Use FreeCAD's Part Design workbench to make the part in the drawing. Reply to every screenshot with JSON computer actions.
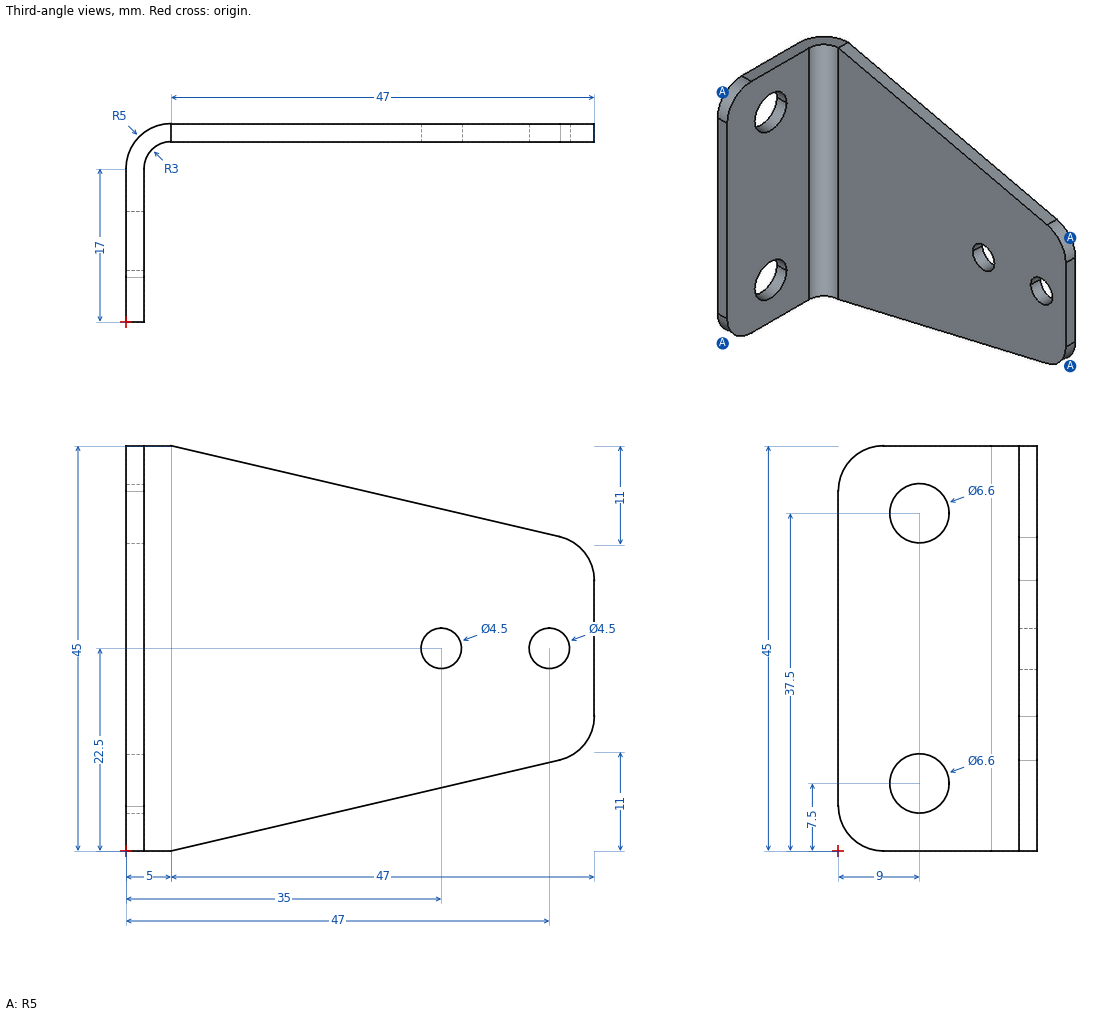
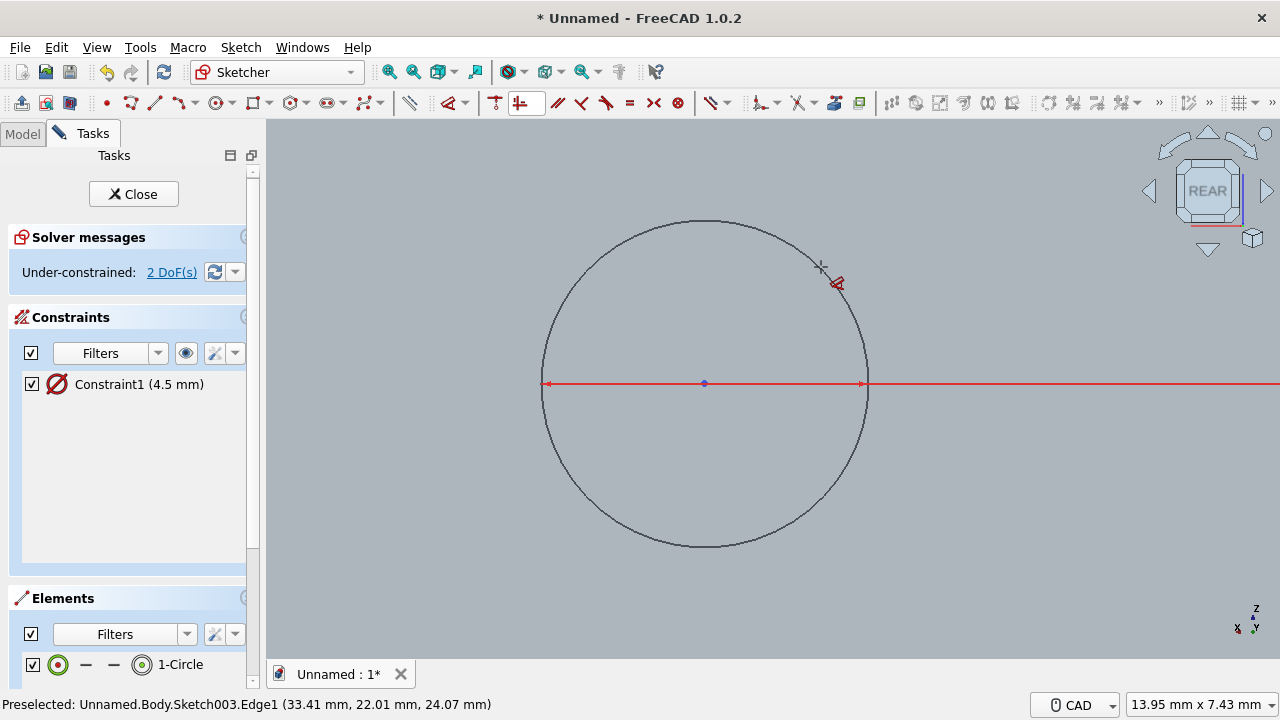
{"action": "left_click", "coordinate": [705, 384]}
{"action": "left_click", "coordinate": [910, 350]}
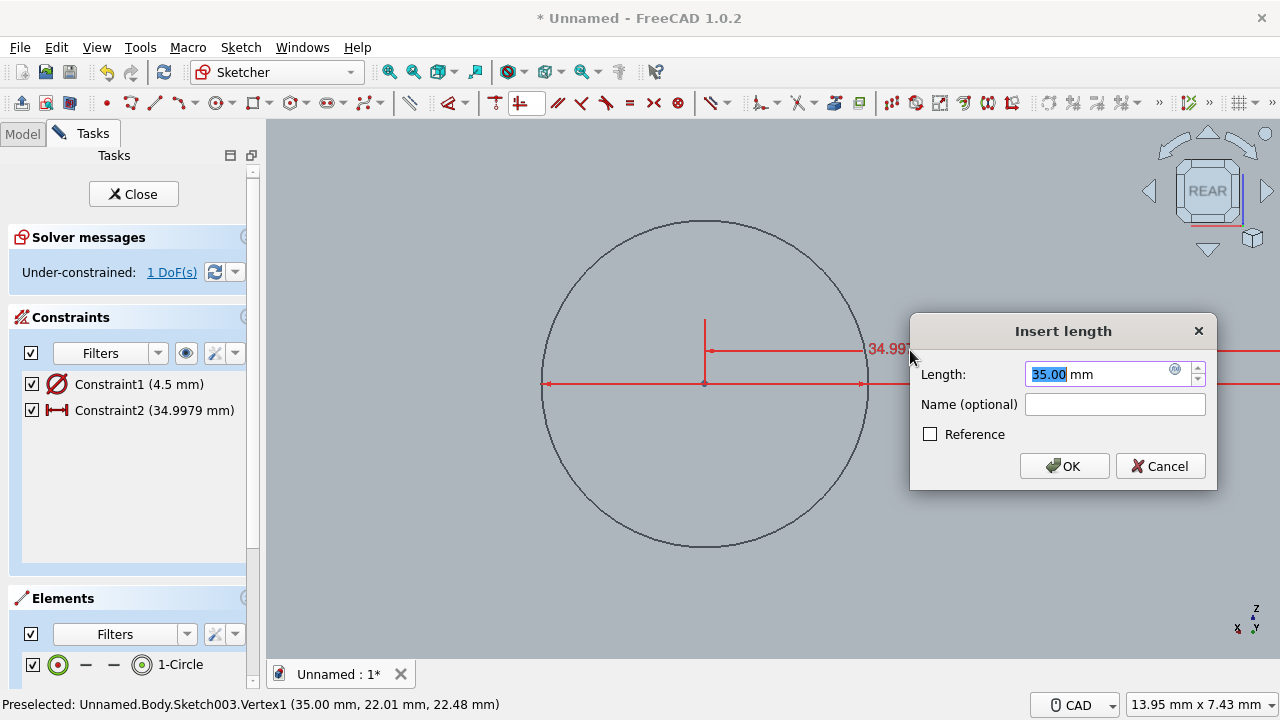
{"action": "type", "text": "35"}
{"action": "key", "text": "Return"}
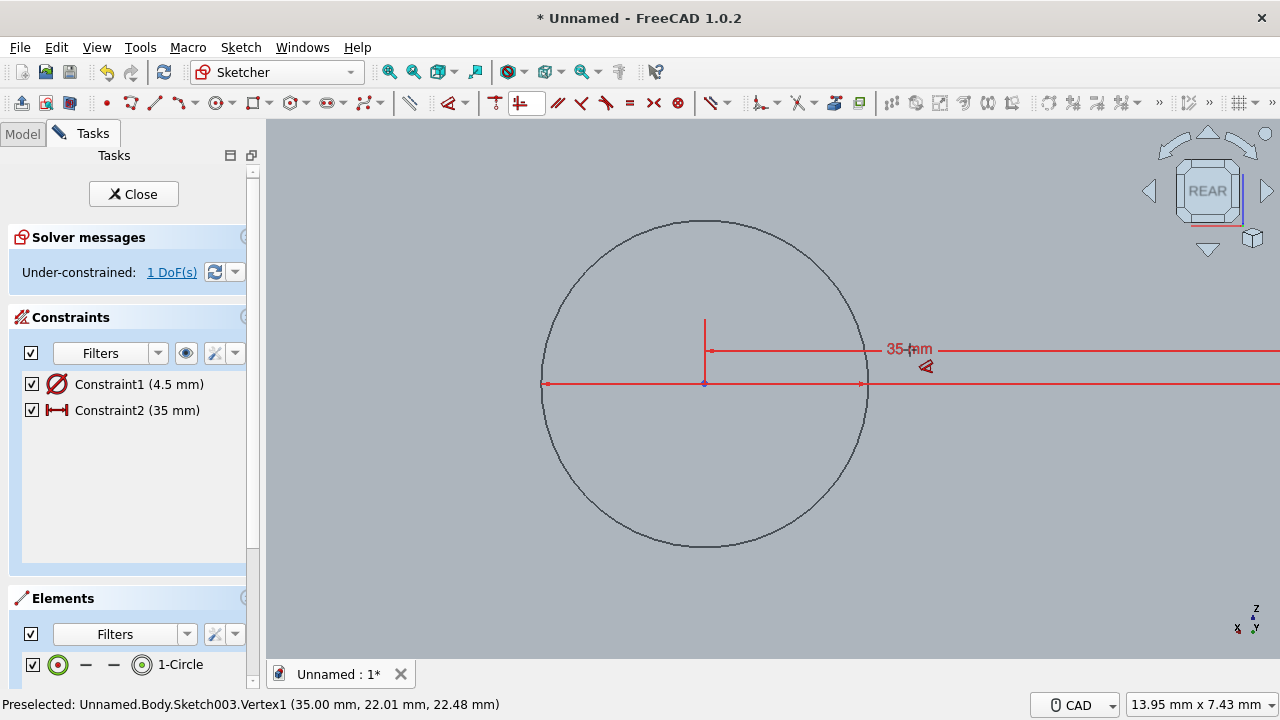
{"action": "left_click", "coordinate": [705, 384]}
{"action": "left_click", "coordinate": [671, 508]}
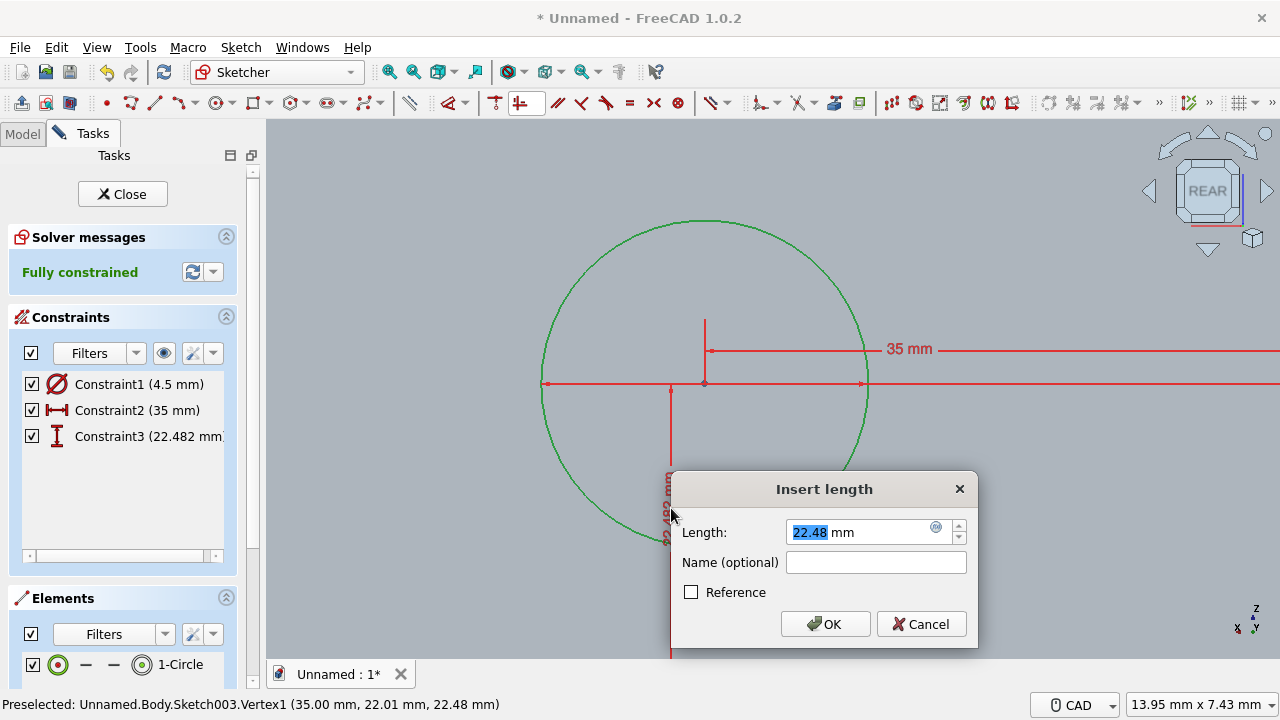
{"action": "type", "text": "22.5"}
{"action": "key", "text": "Return"}
{"action": "key", "text": "Escape"}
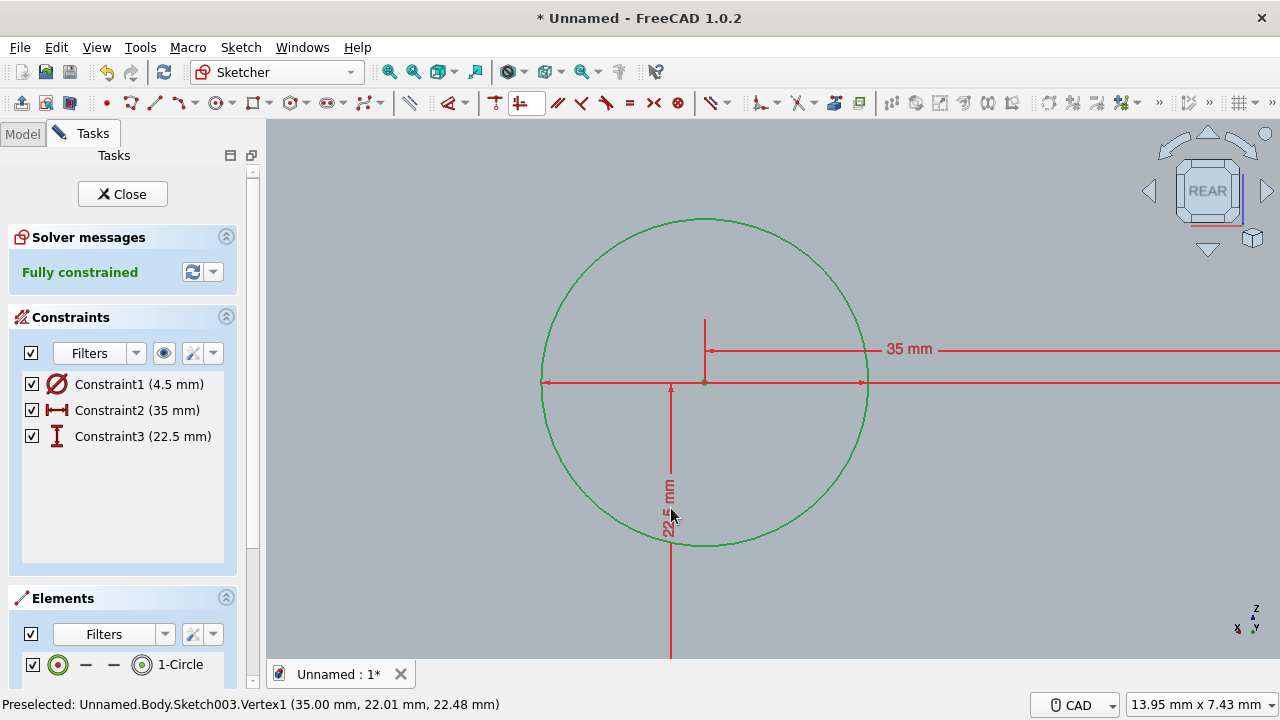
{"action": "left_click", "coordinate": [123, 194]}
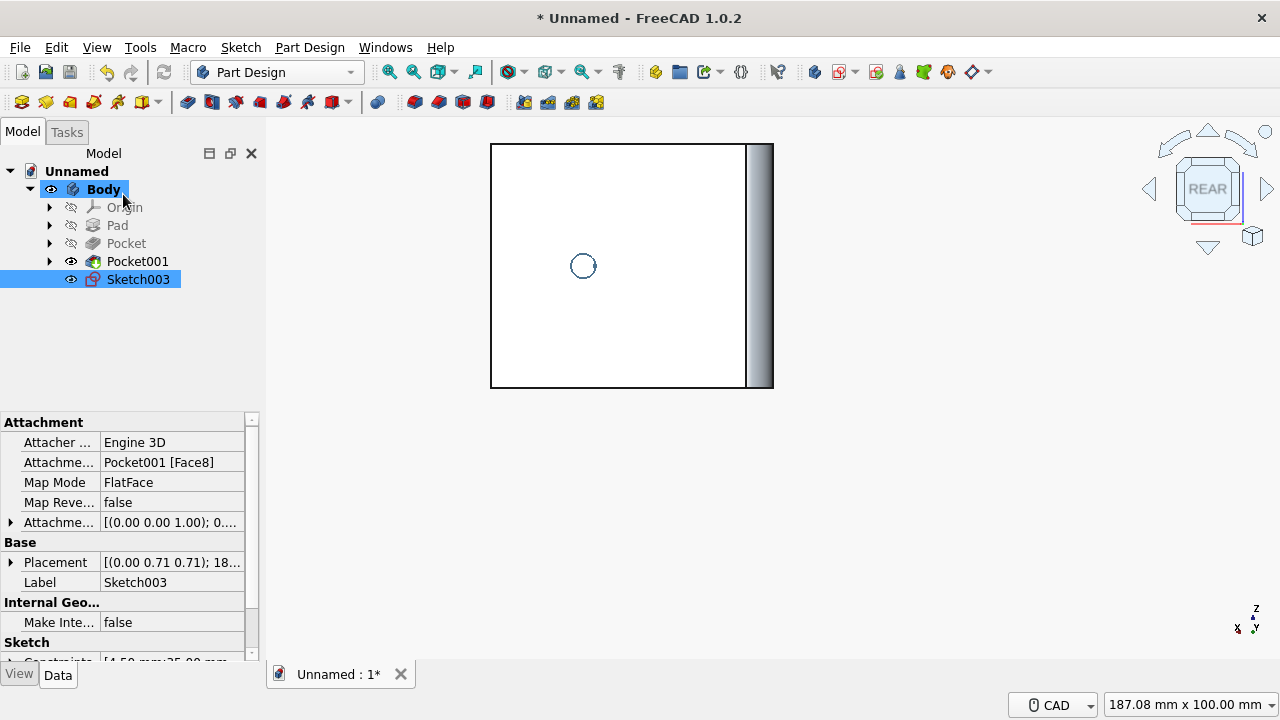
{"action": "left_click", "coordinate": [188, 102]}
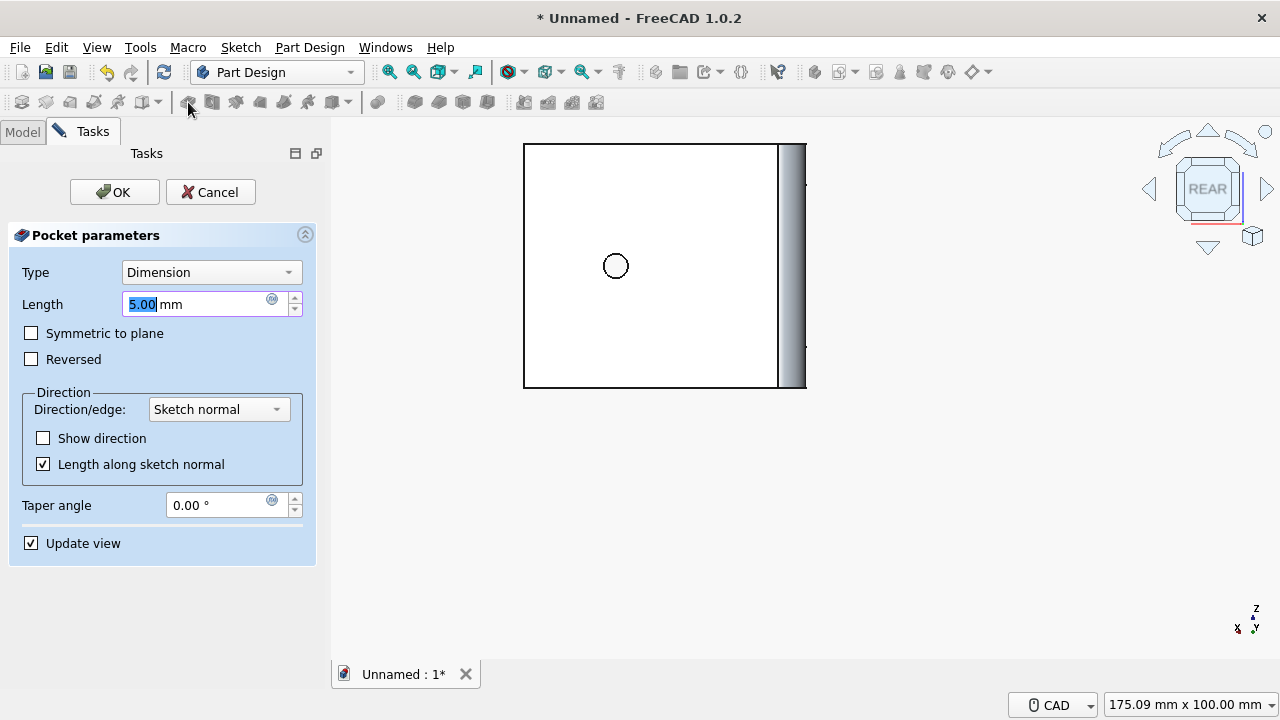
{"action": "left_click", "coordinate": [212, 272]}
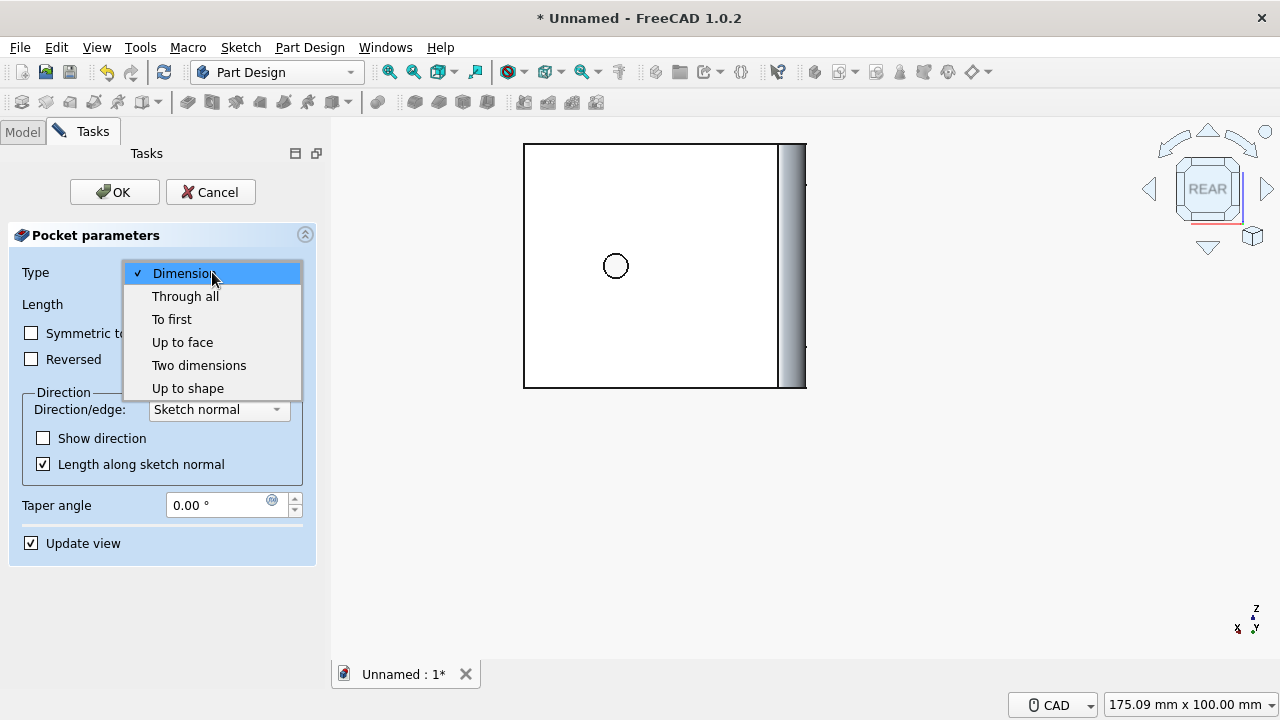
{"action": "left_click", "coordinate": [212, 320]}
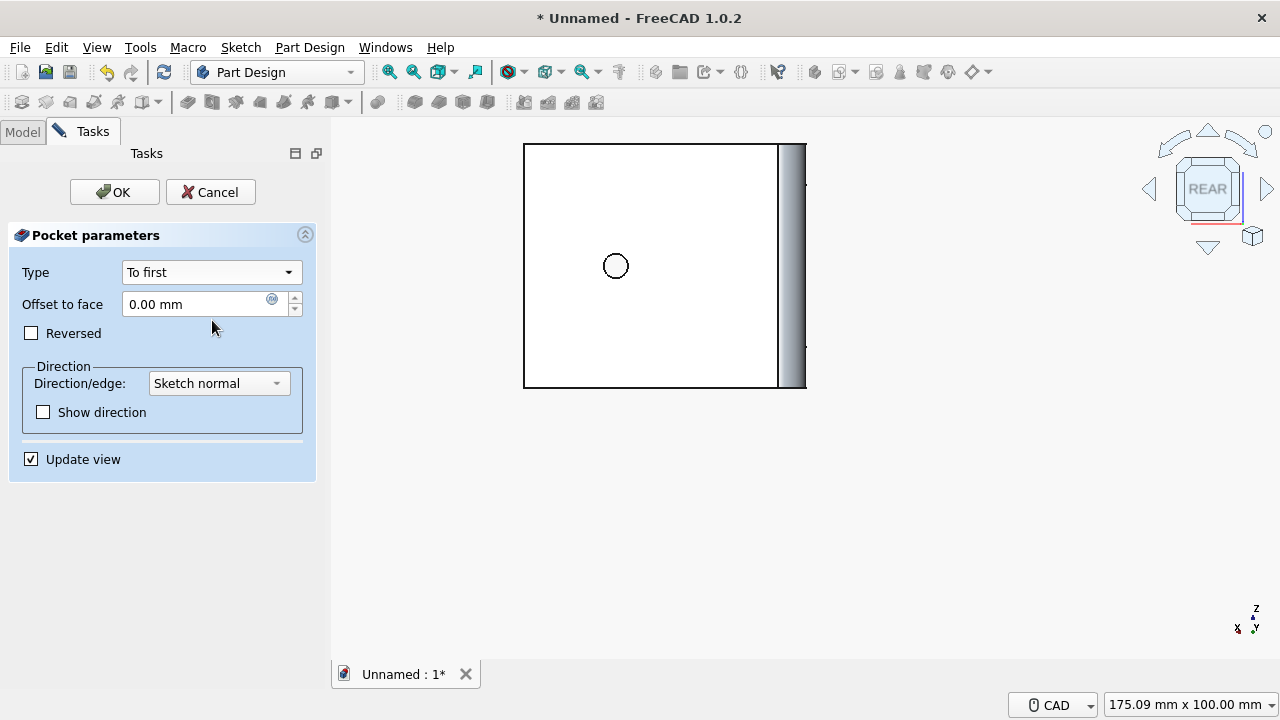
{"action": "left_click", "coordinate": [115, 192]}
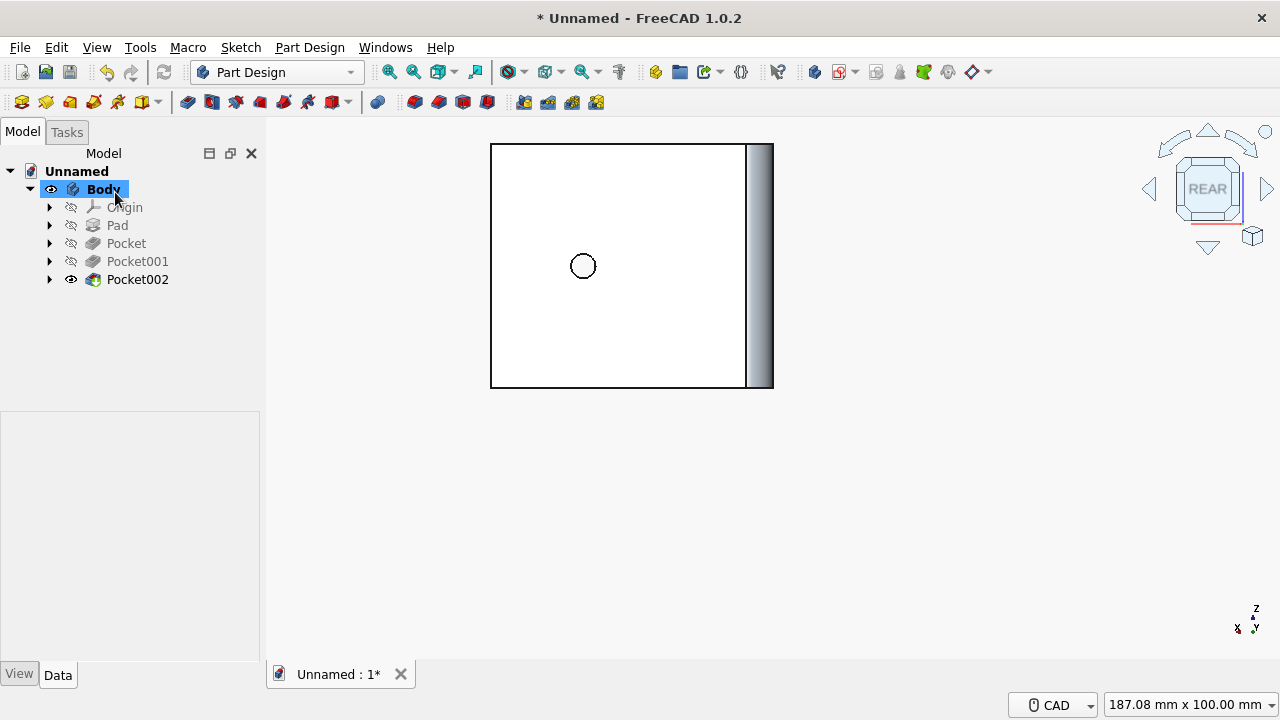
{"action": "left_click", "coordinate": [655, 230]}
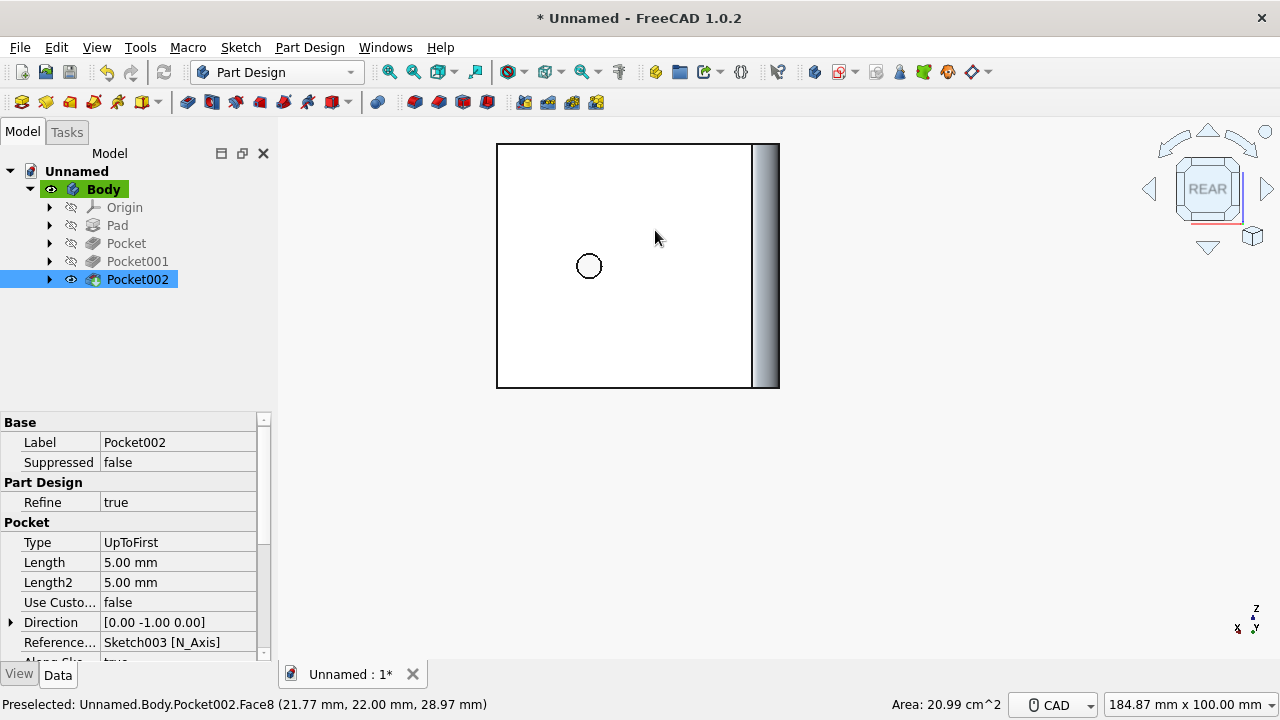
{"action": "left_click", "coordinate": [840, 72]}